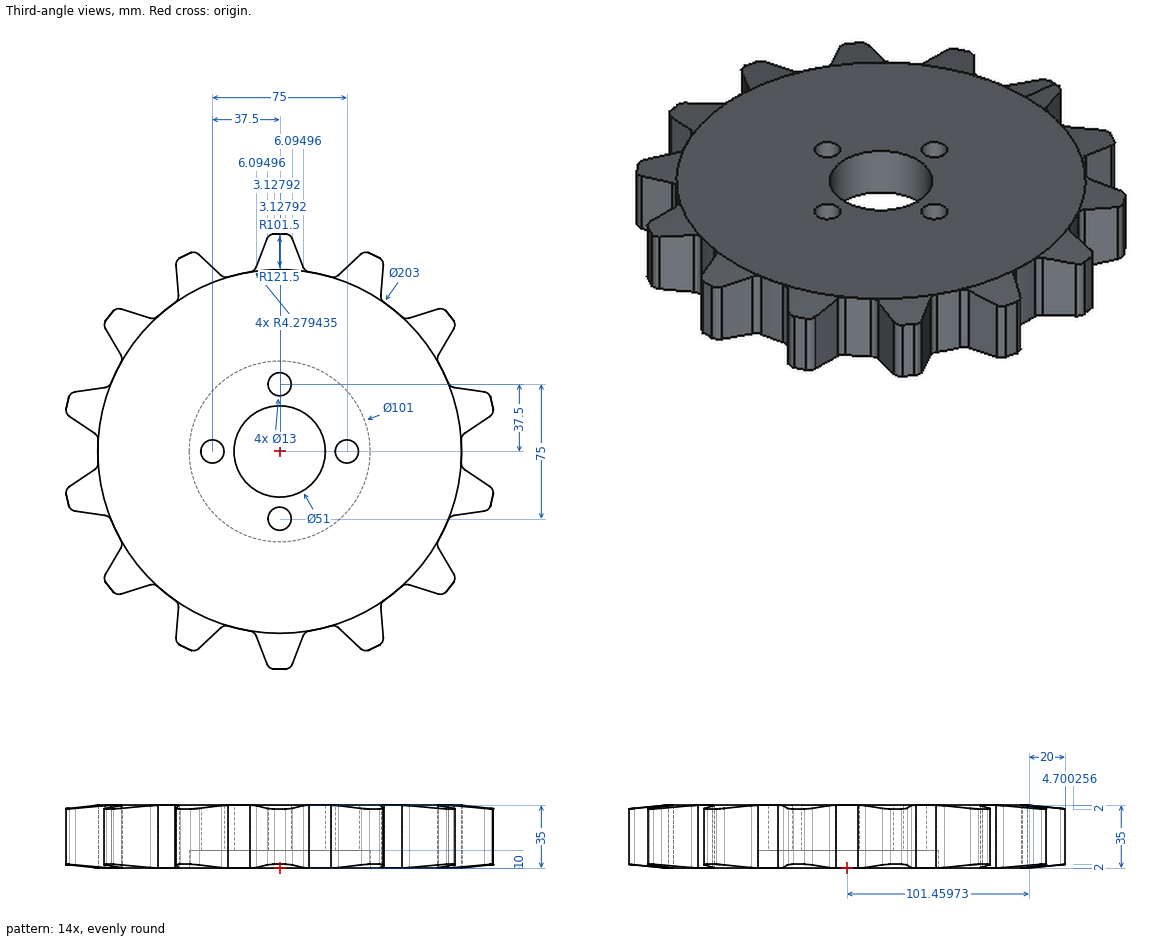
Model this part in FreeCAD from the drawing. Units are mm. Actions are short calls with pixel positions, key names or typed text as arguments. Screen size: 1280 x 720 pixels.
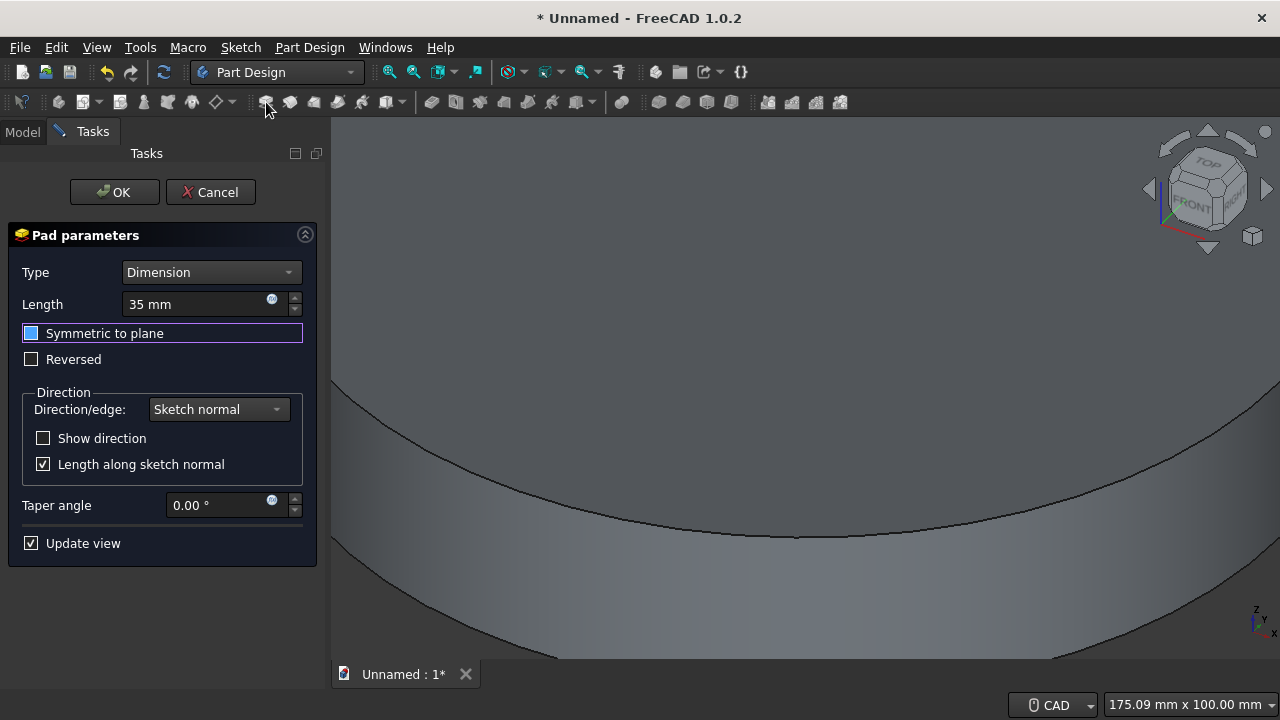
click(115, 192)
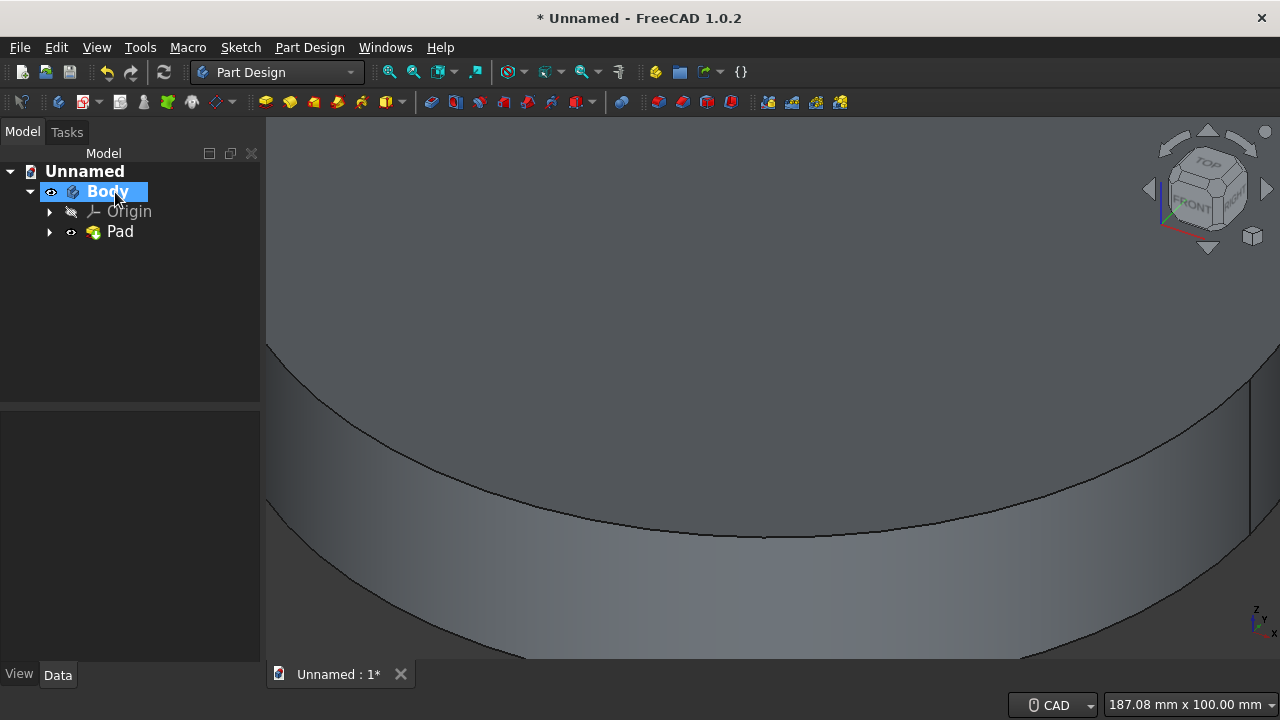
click(390, 72)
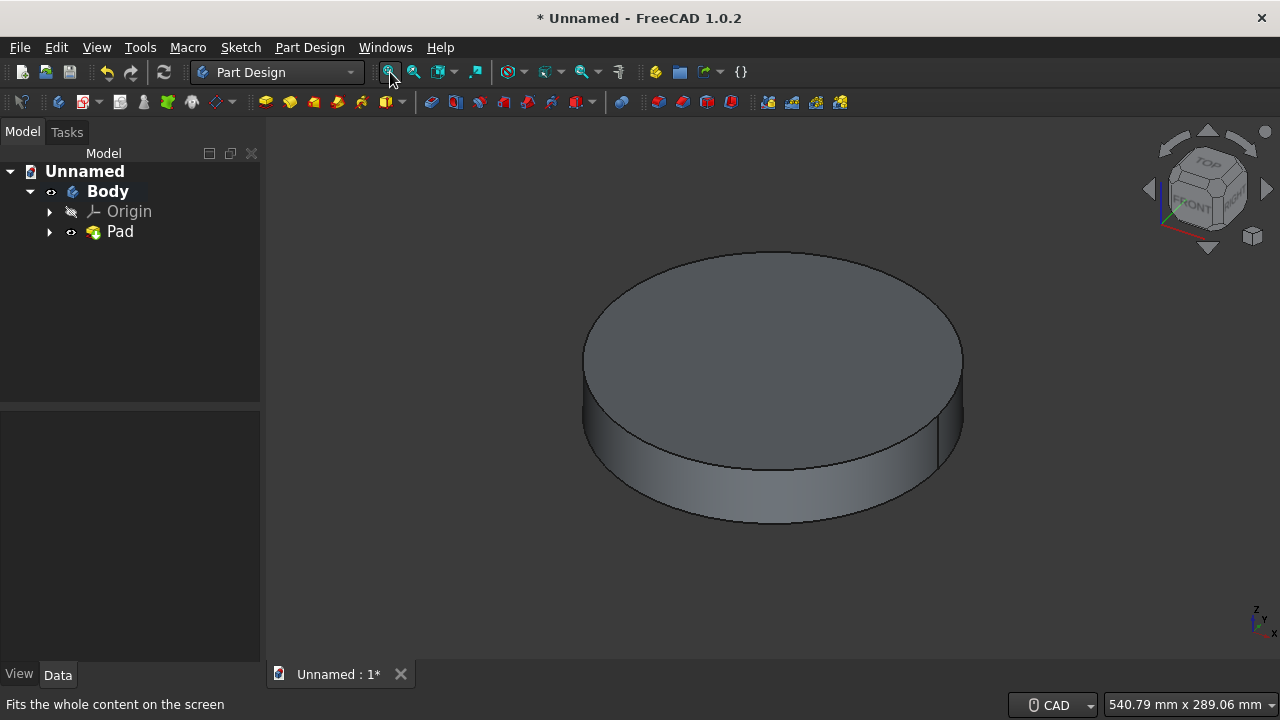
click(84, 102)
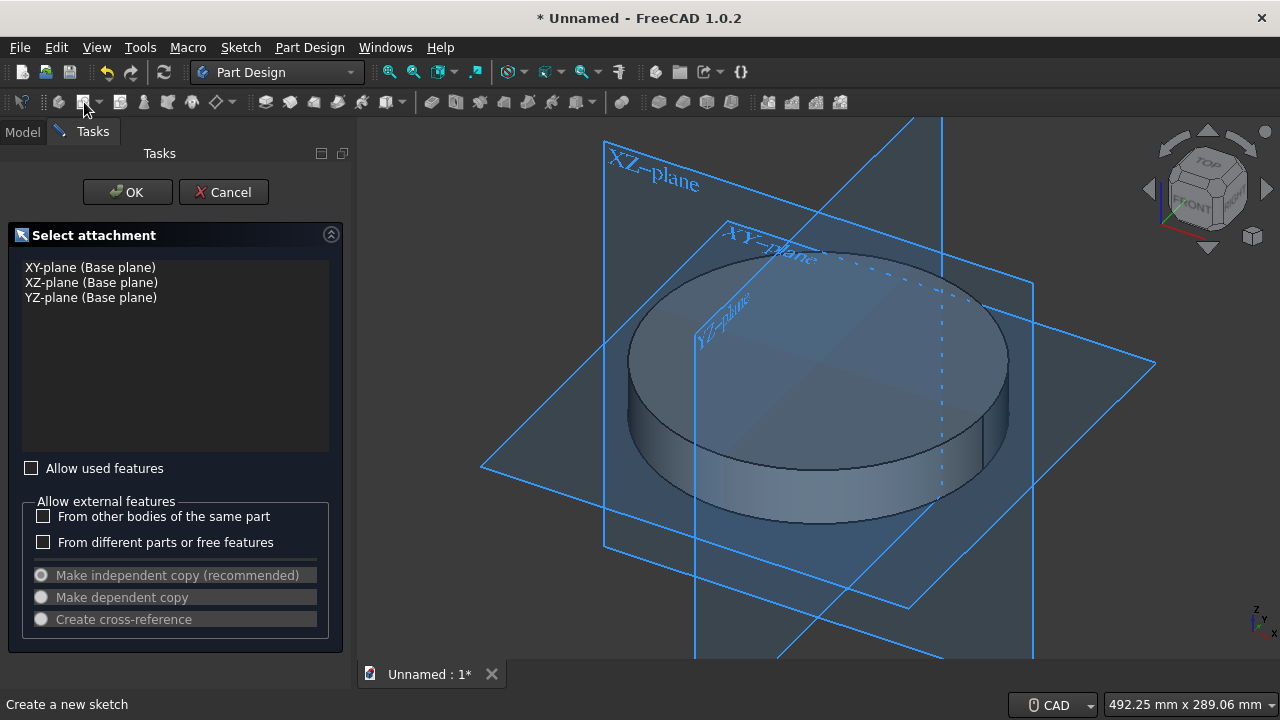
click(82, 268)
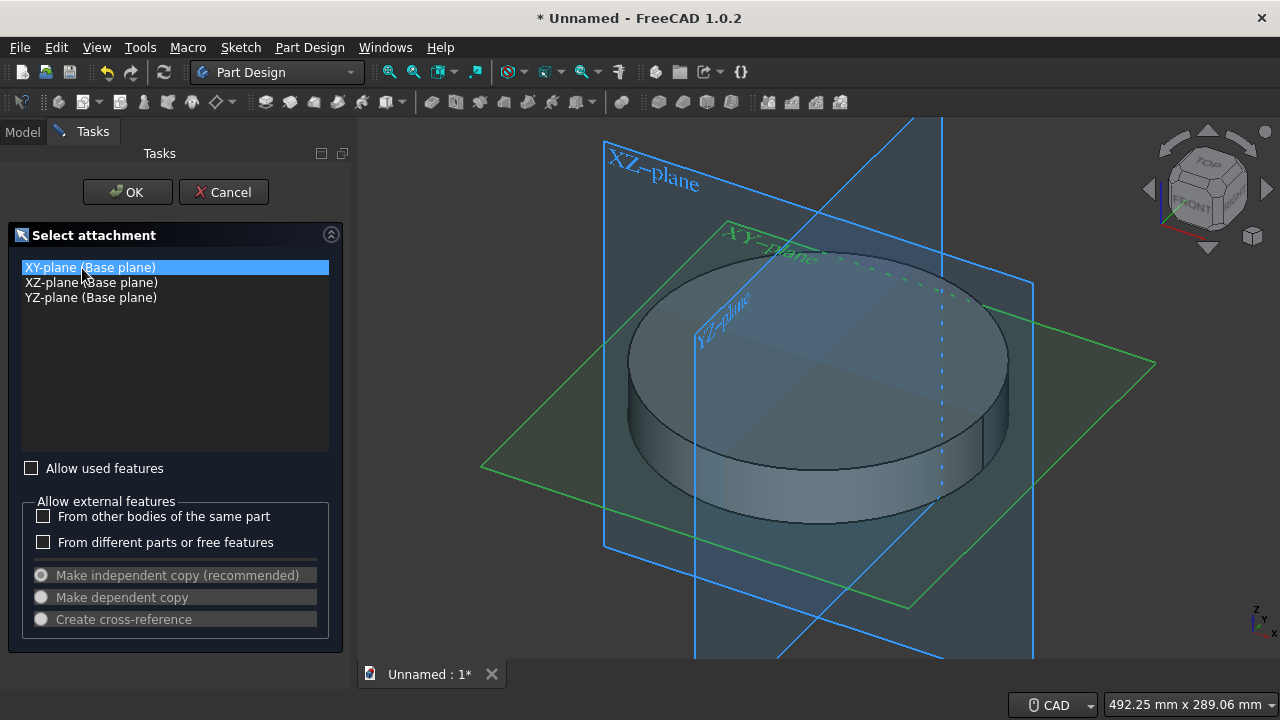
click(128, 192)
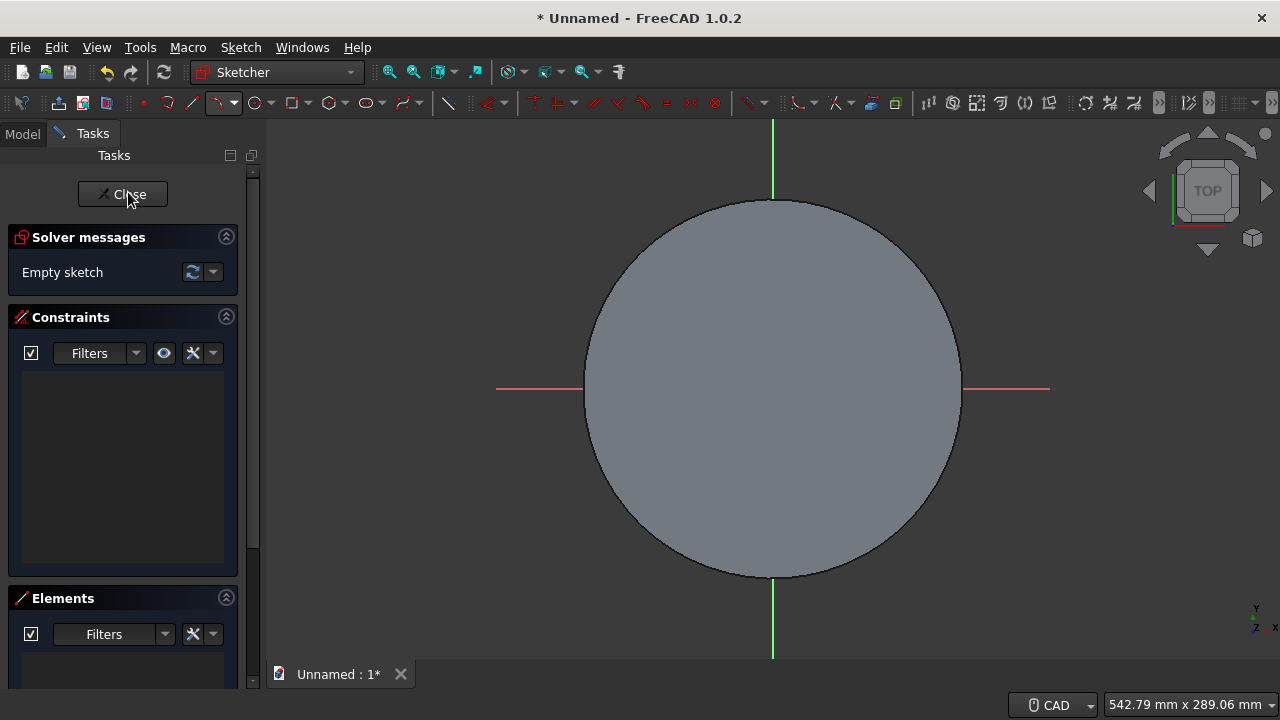
click(108, 104)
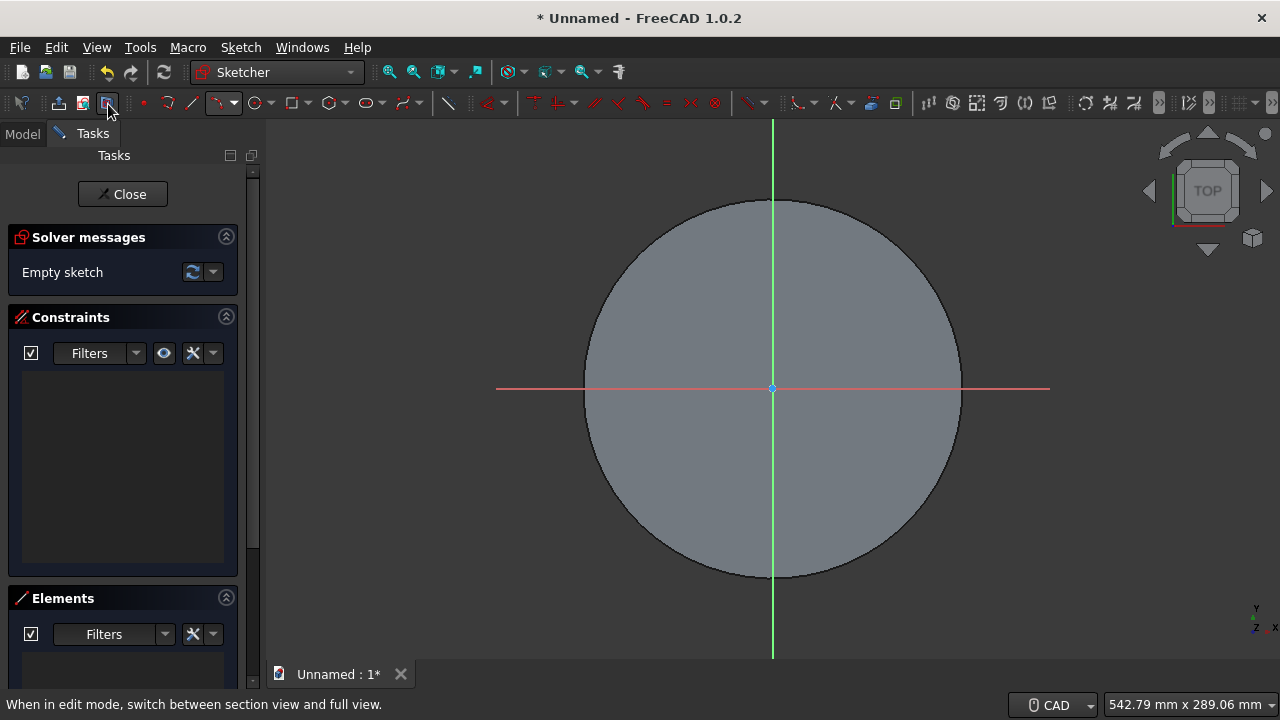
scroll(781, 156, up, 11)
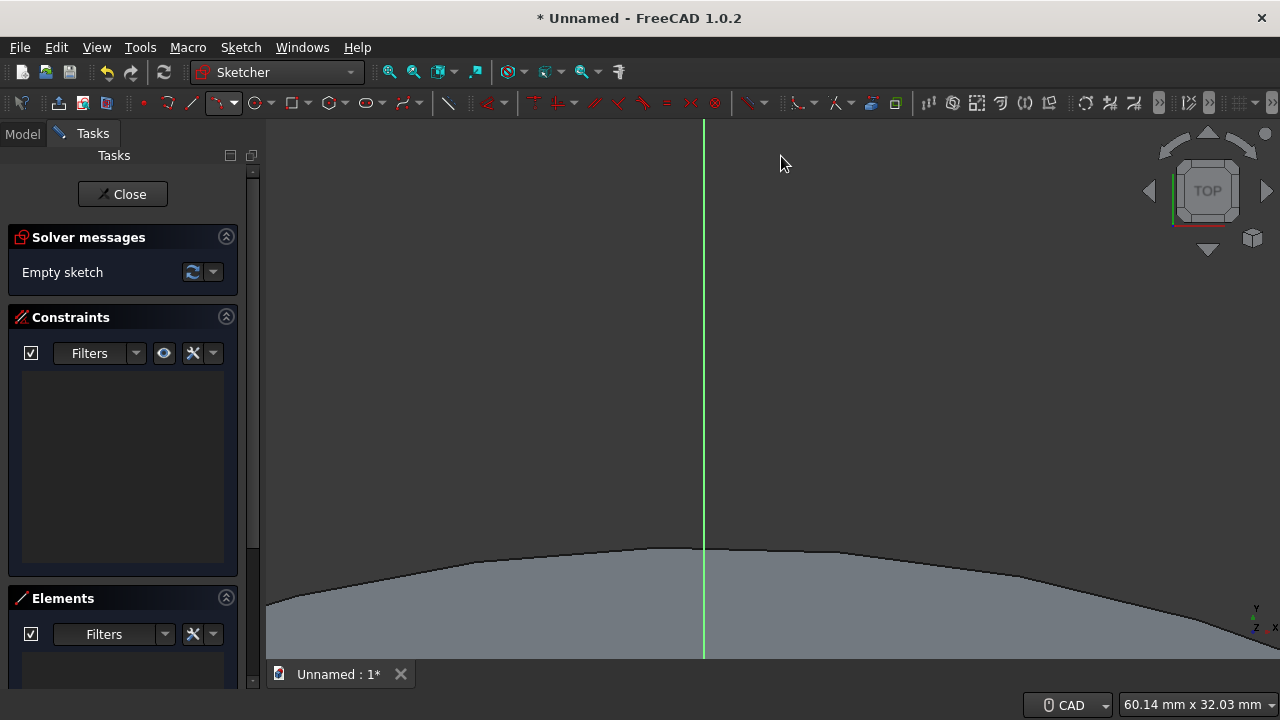
click(192, 104)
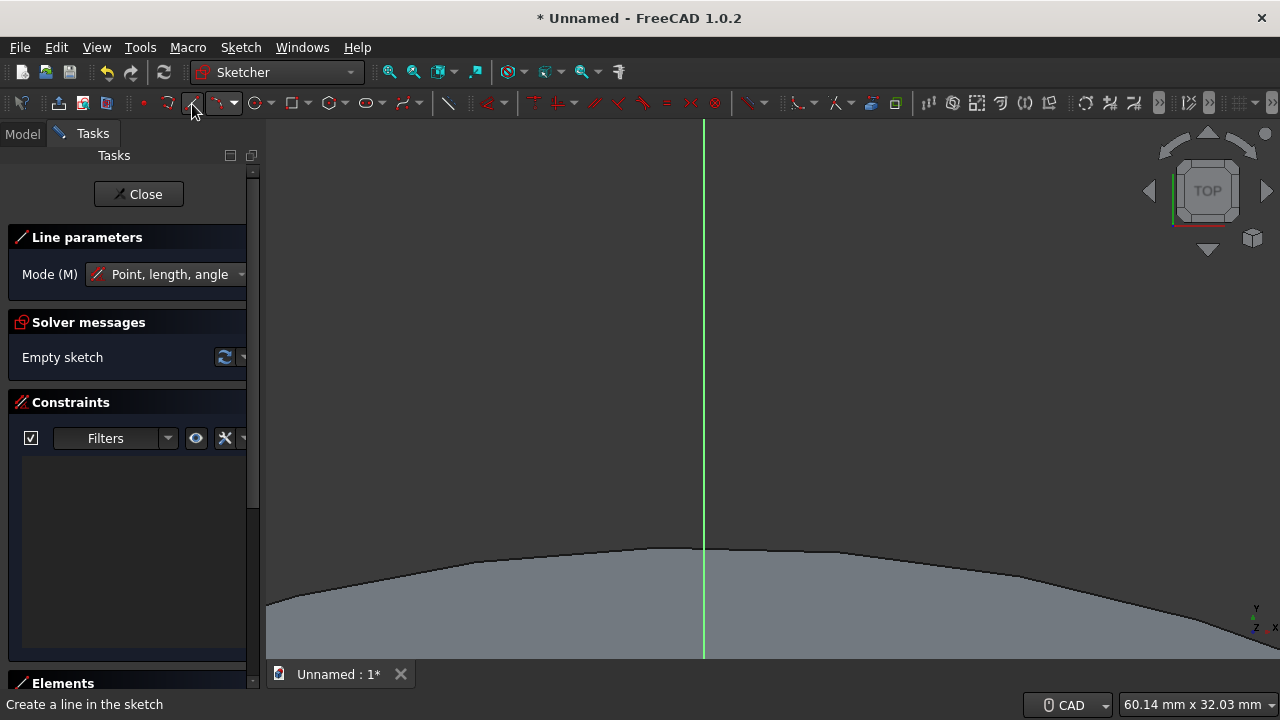
click(585, 257)
click(483, 524)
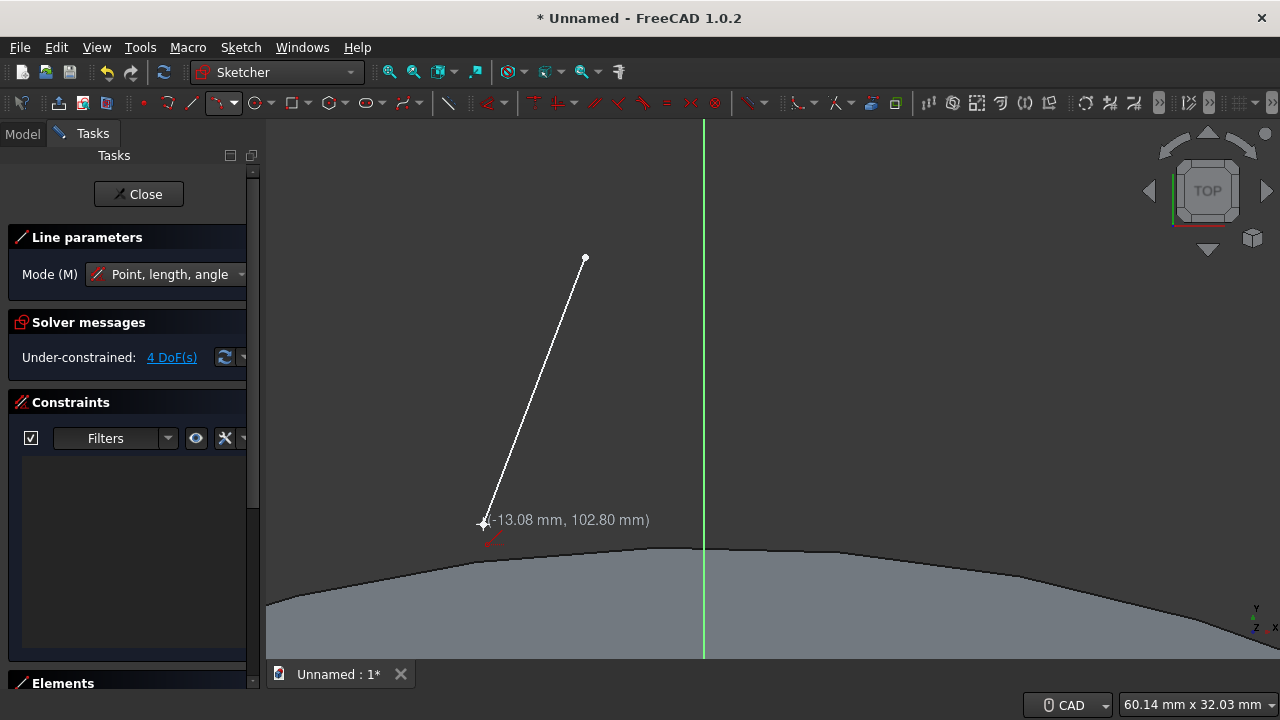
click(924, 524)
click(822, 257)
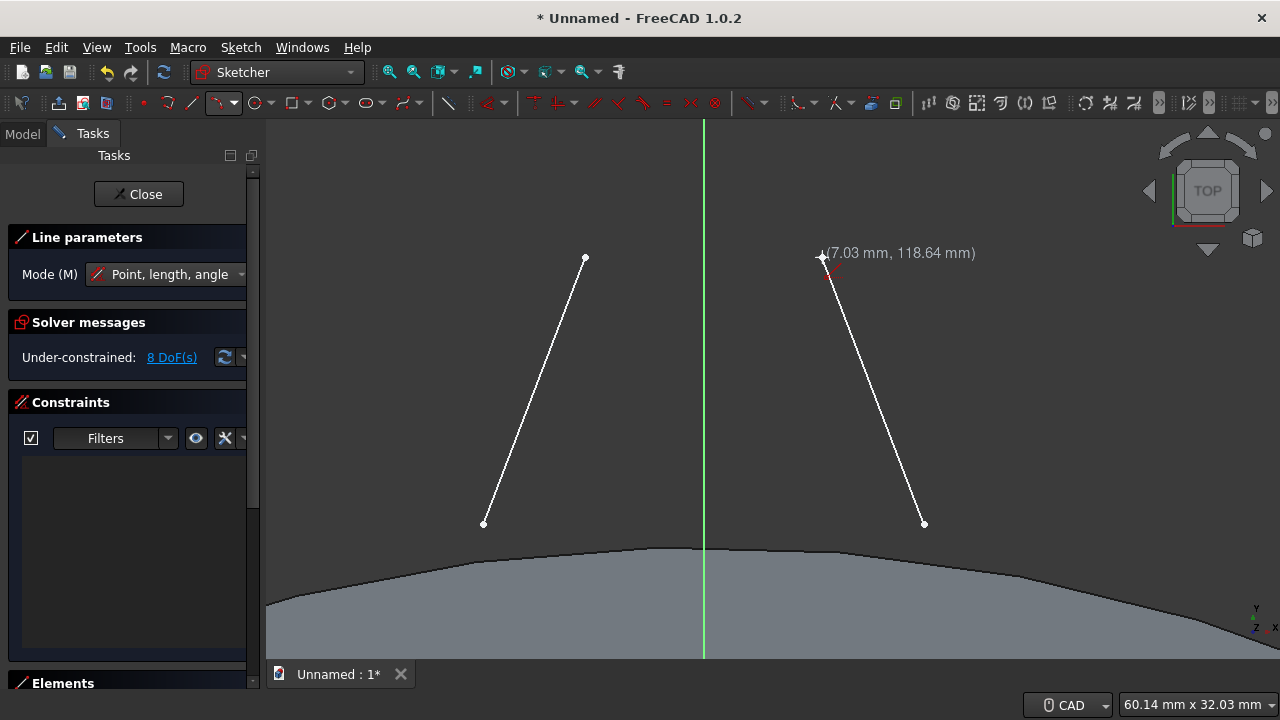
click(218, 104)